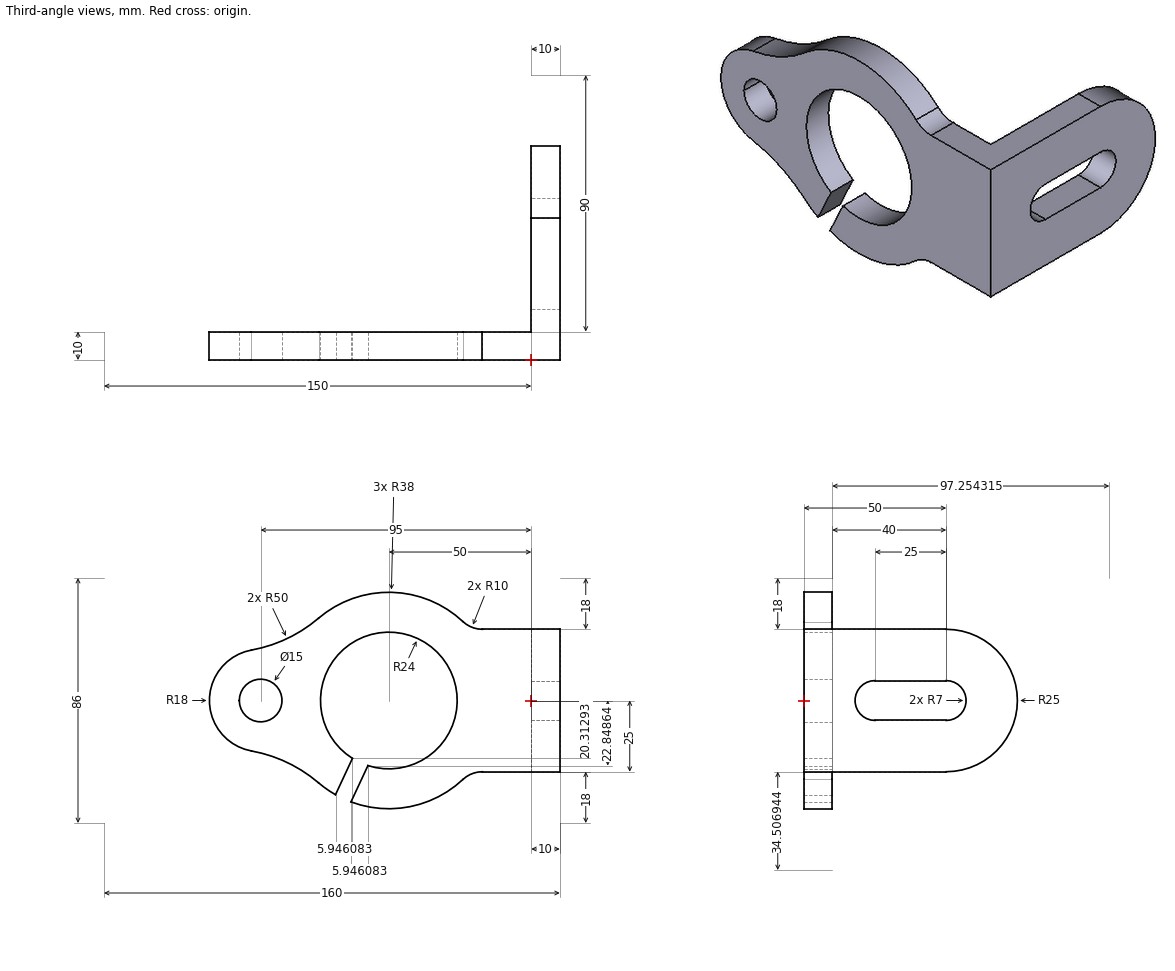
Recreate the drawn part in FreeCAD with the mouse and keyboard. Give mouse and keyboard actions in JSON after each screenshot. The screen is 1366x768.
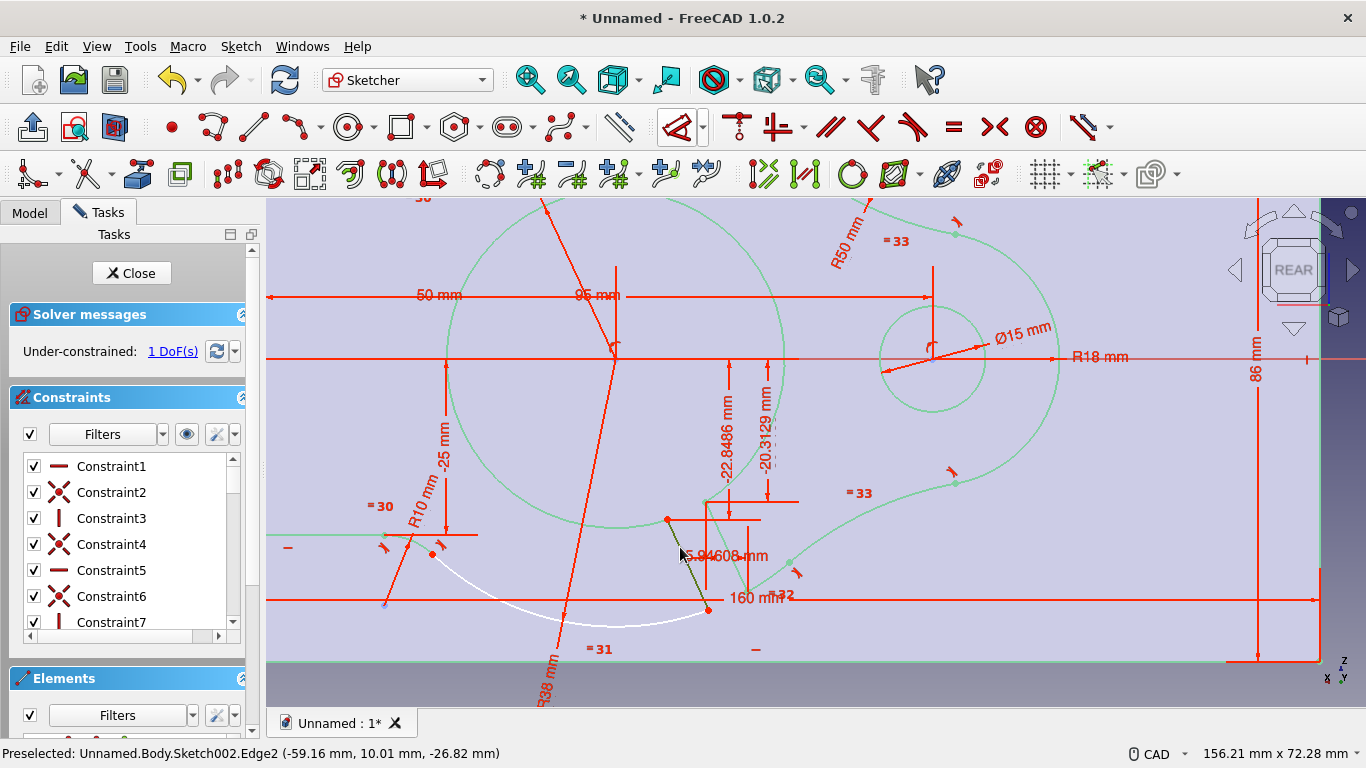
{"action": "key", "text": "l"}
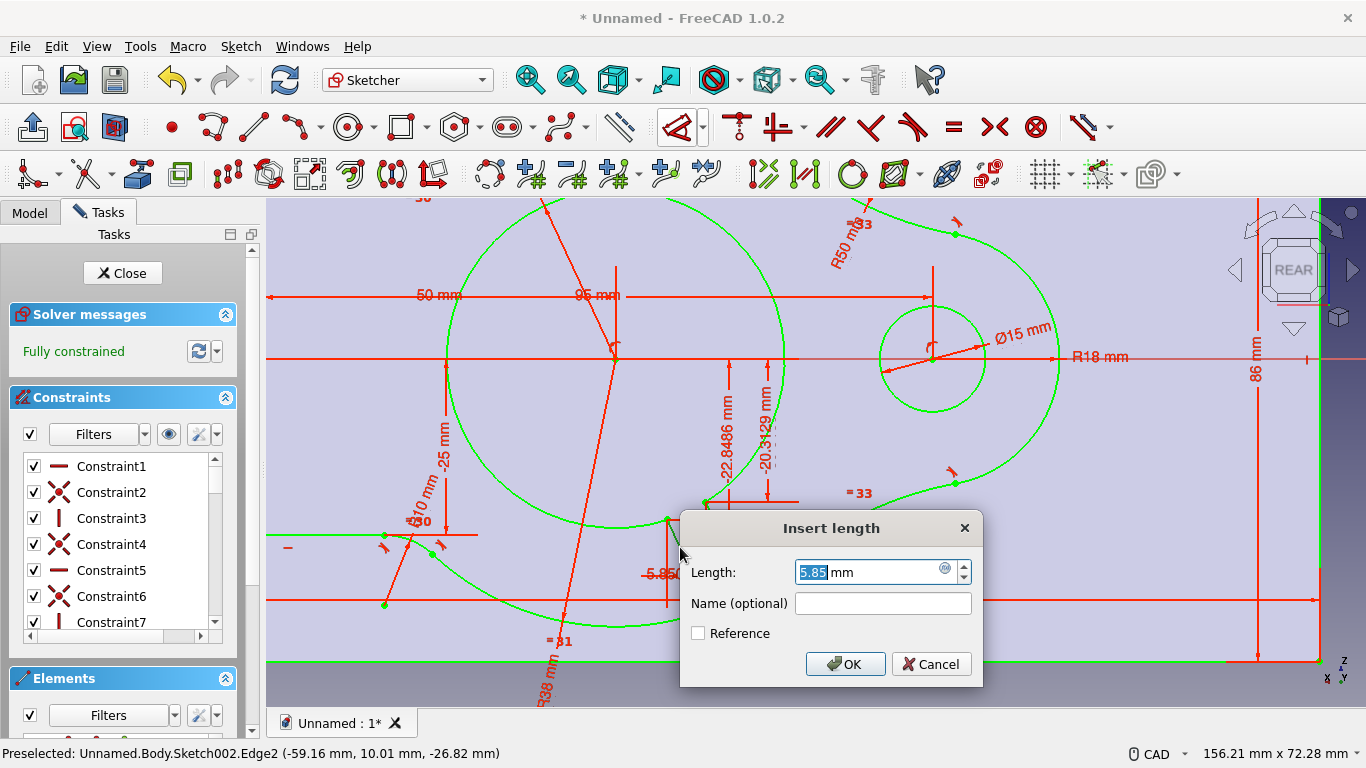
{"action": "type", "text": "5.946083"}
{"action": "key", "text": "Return"}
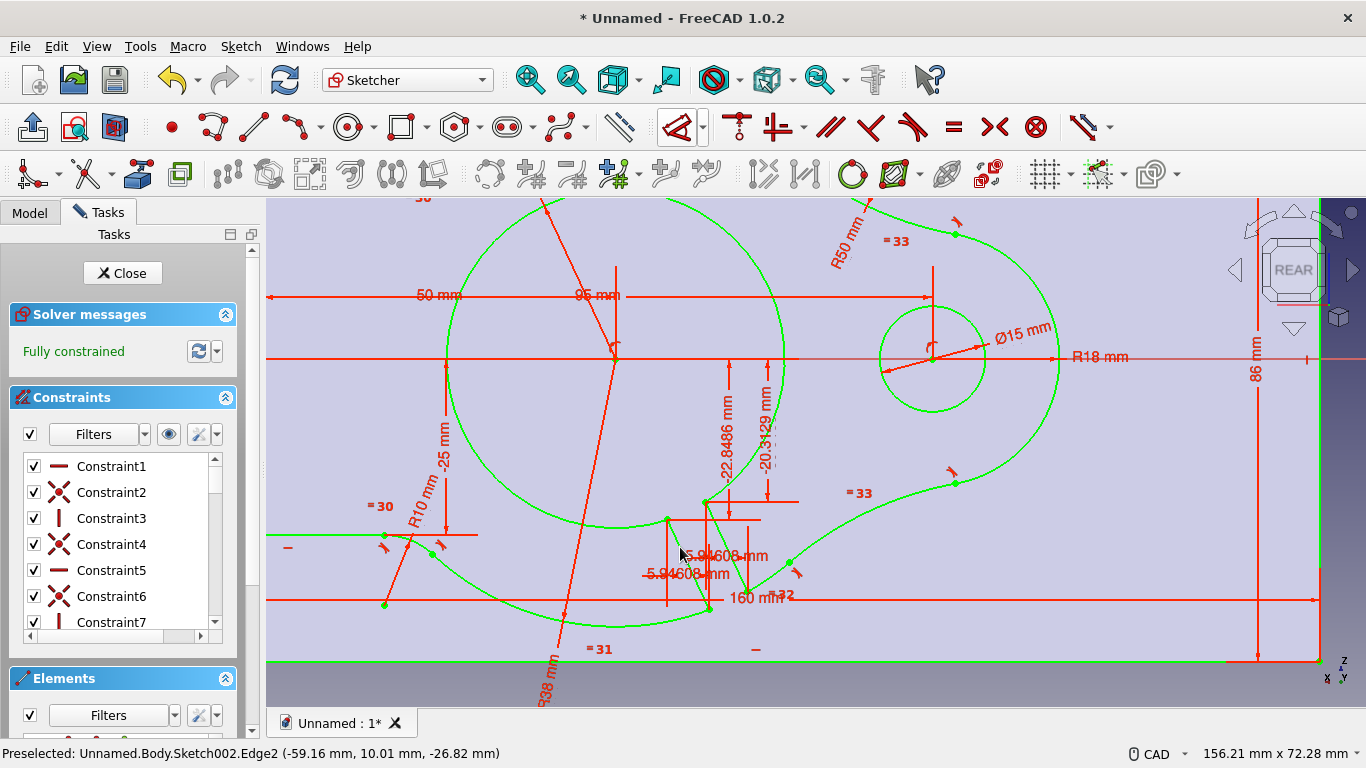
{"action": "left_click", "coordinate": [123, 273]}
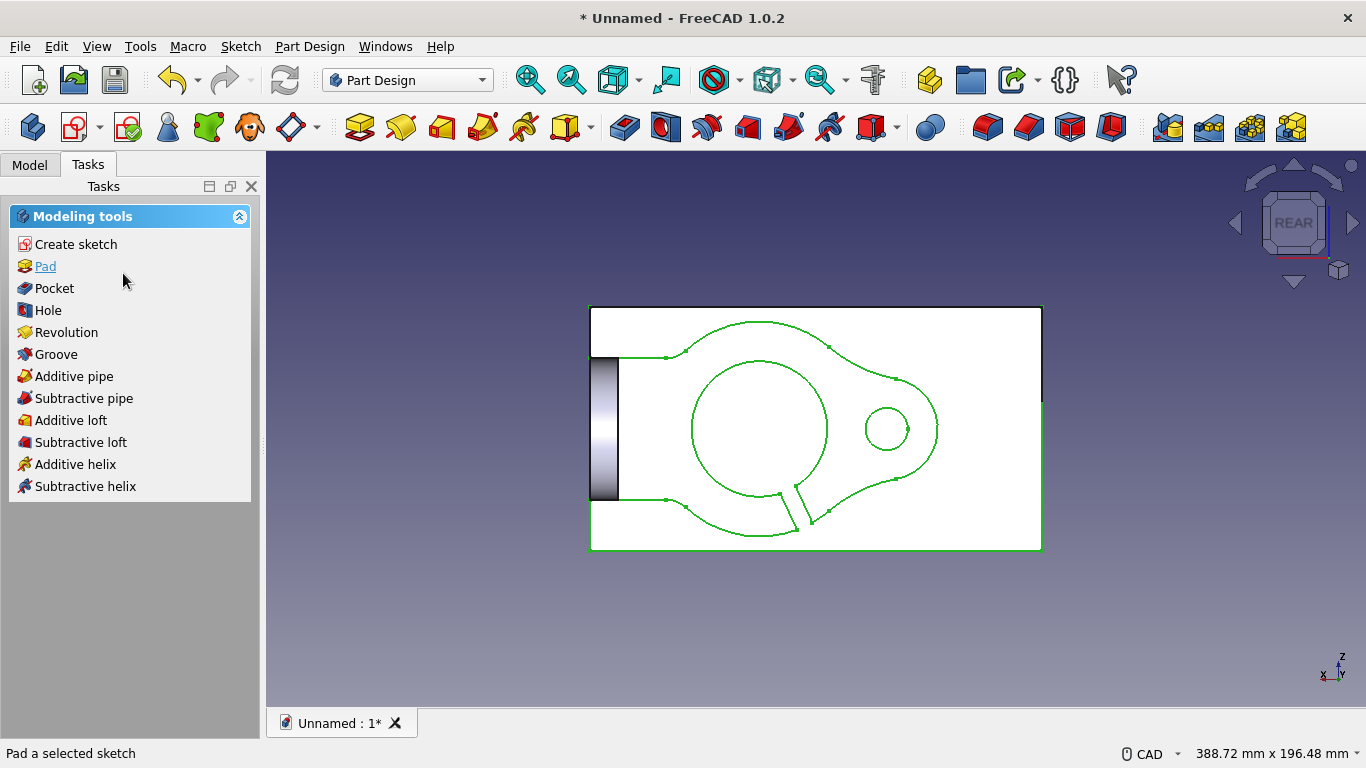
{"action": "left_click", "coordinate": [625, 128]}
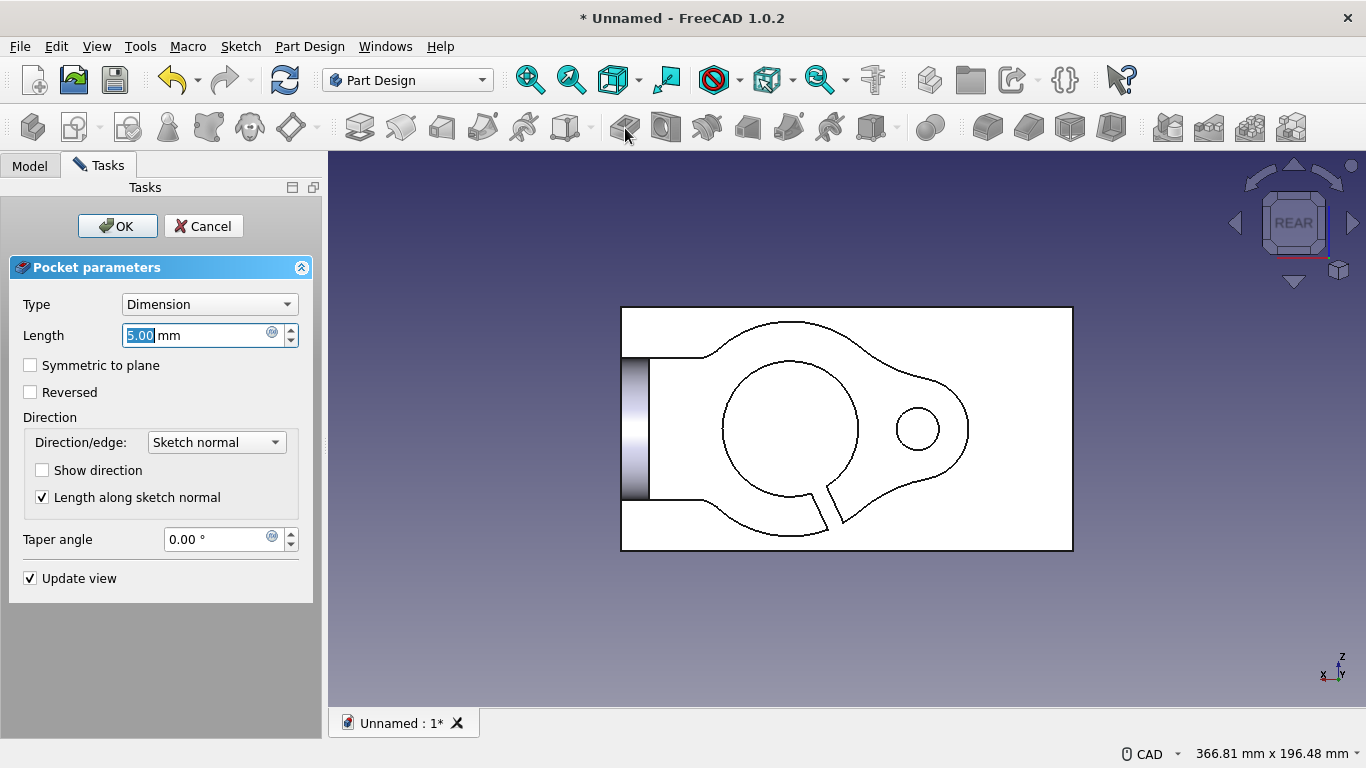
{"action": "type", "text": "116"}
{"action": "key", "text": "Tab"}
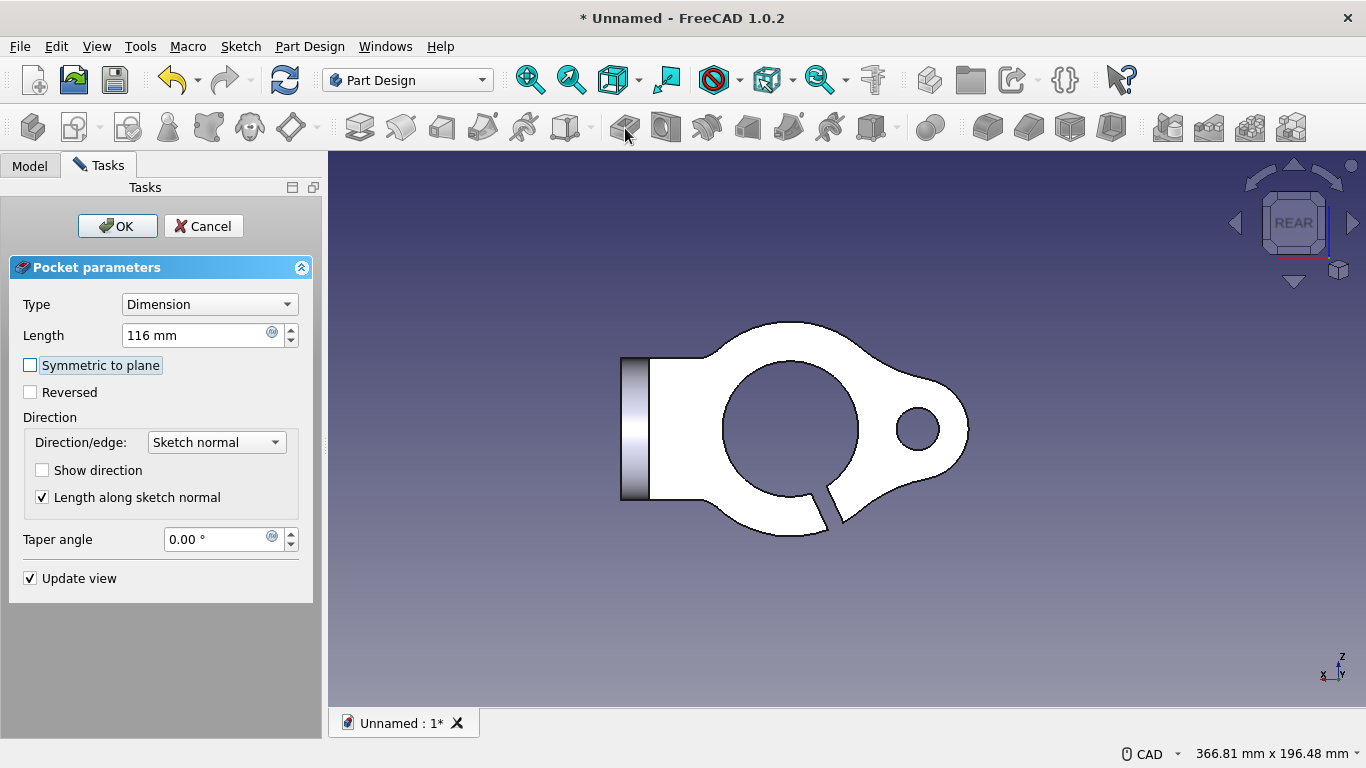
{"action": "left_click", "coordinate": [118, 226]}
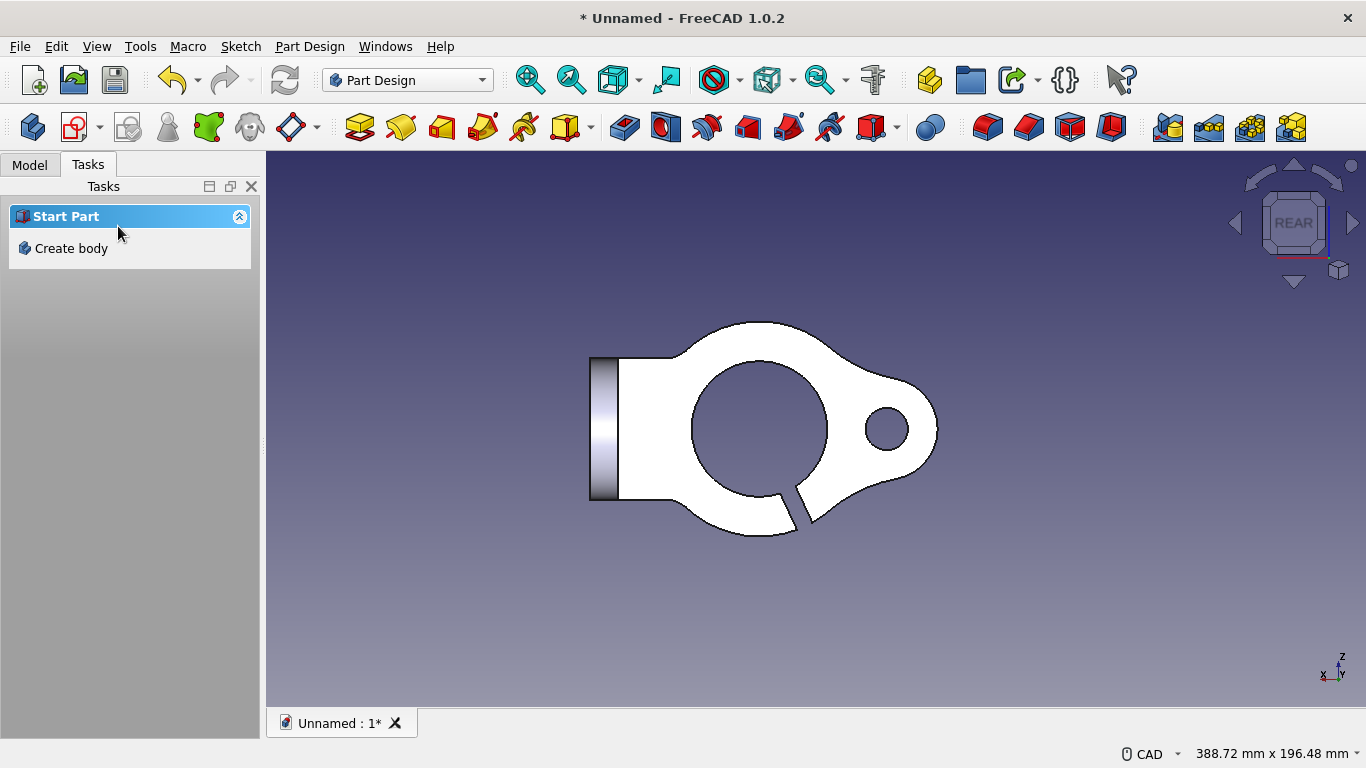
{"action": "key", "text": "0"}